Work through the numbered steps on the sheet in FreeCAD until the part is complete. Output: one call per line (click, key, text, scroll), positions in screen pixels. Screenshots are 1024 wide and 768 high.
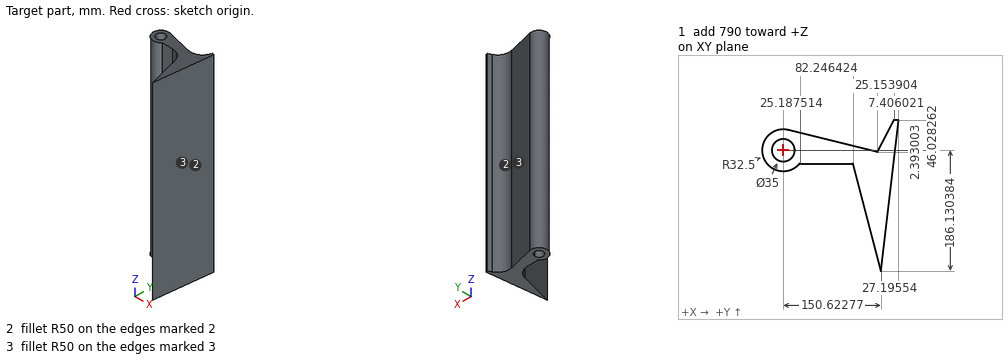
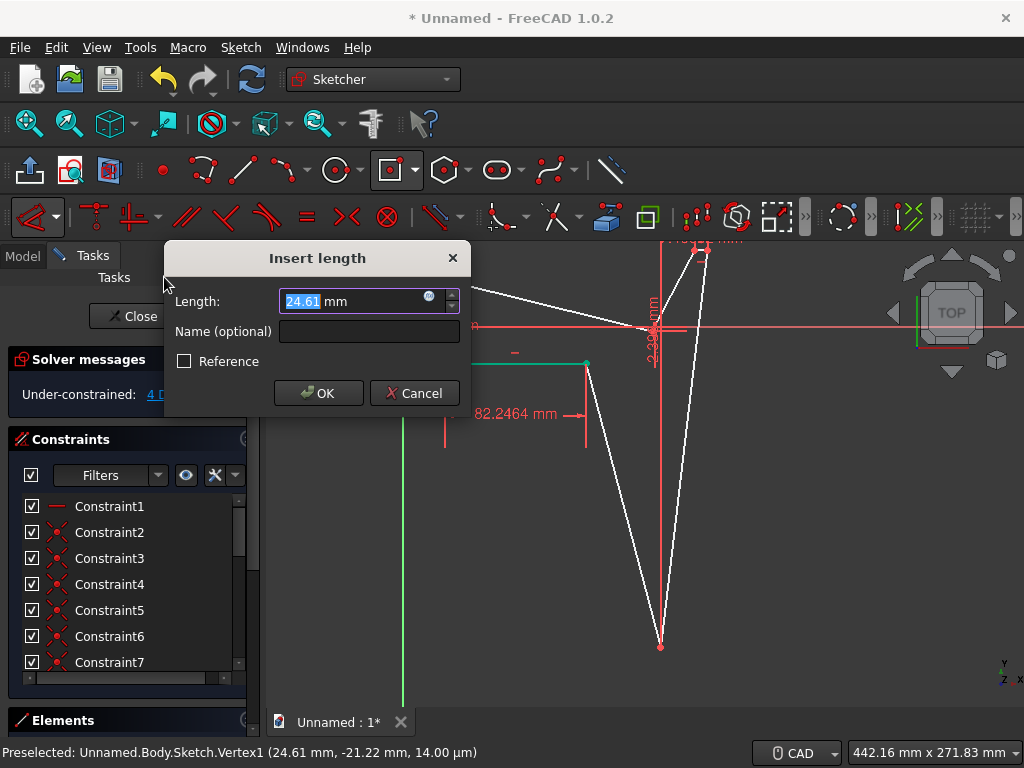
text(25.187514)
key(Return)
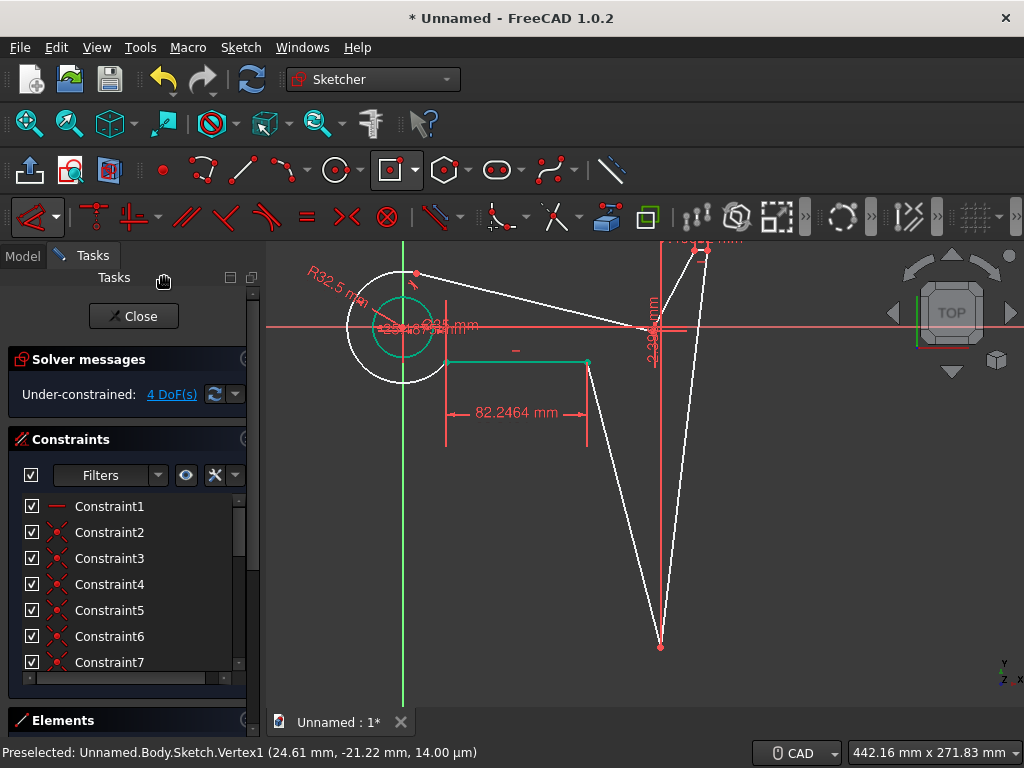
click(661, 647)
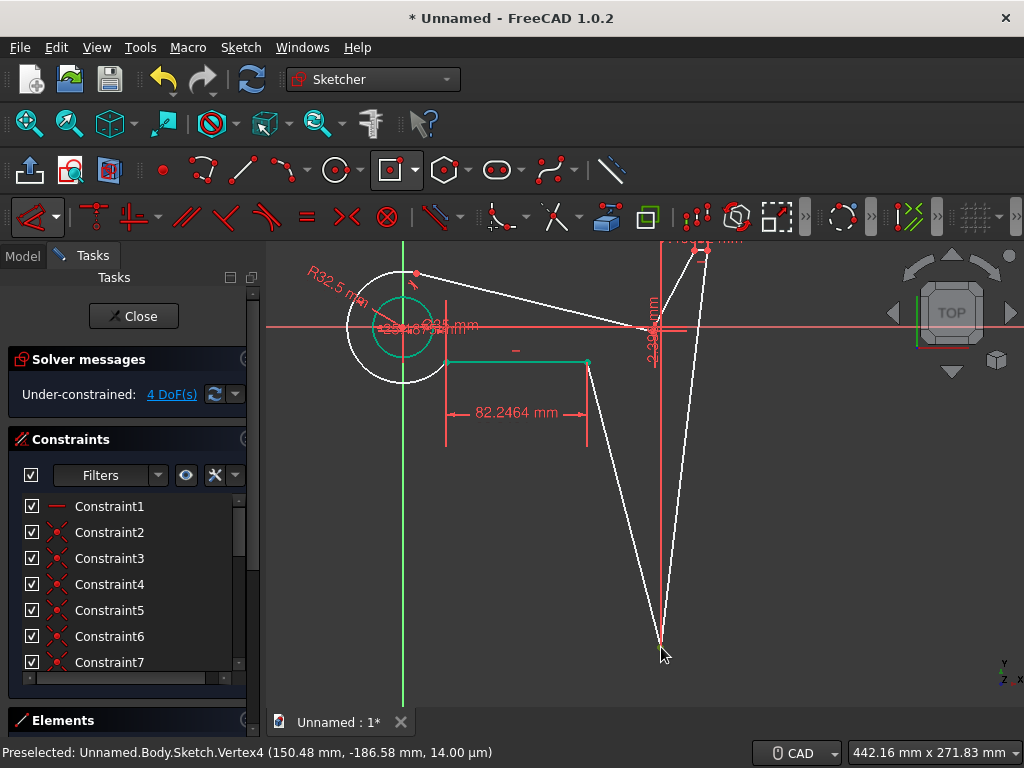
key(l)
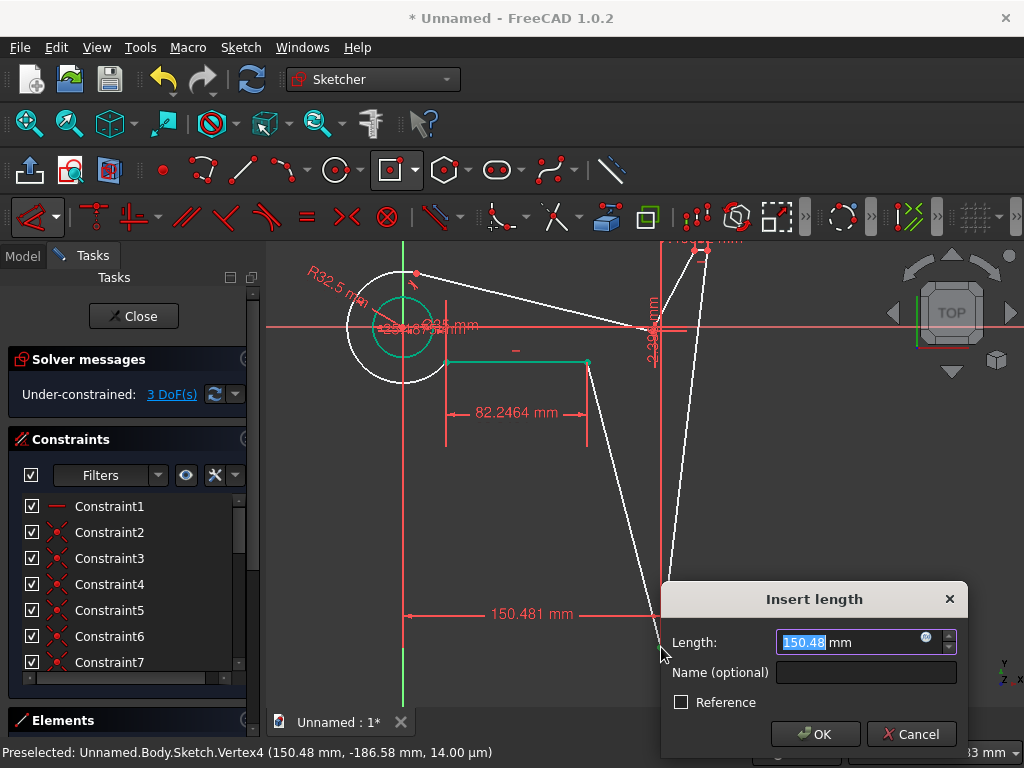
text(150.62277)
key(Return)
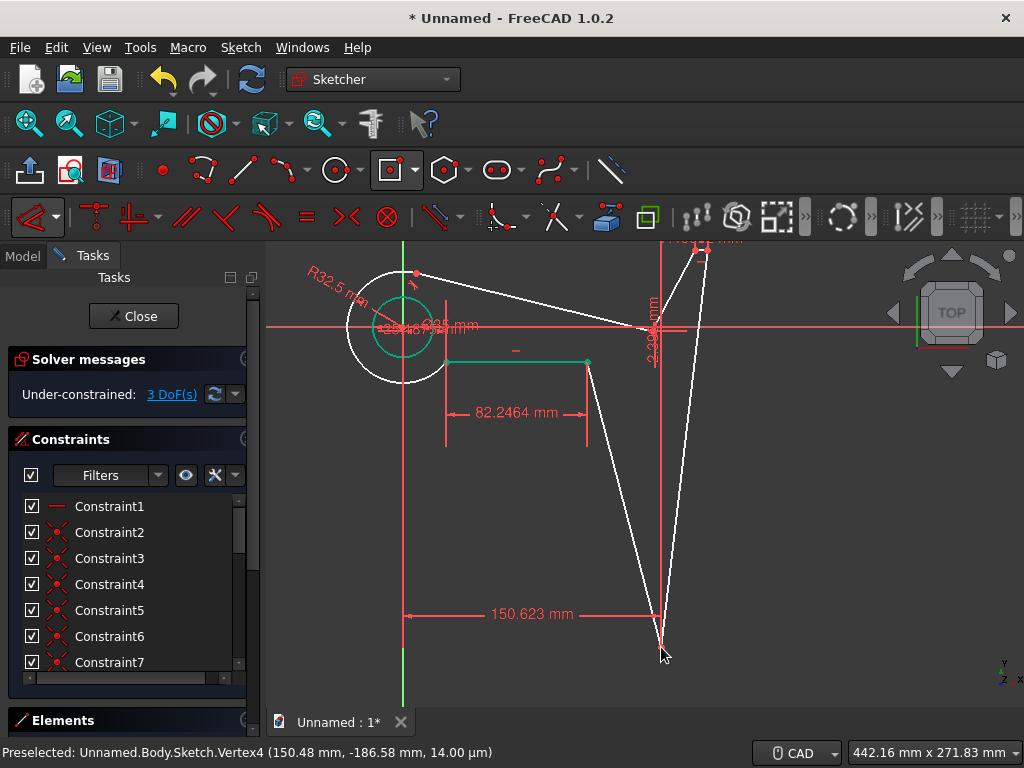
scroll(673, 528, down, 2)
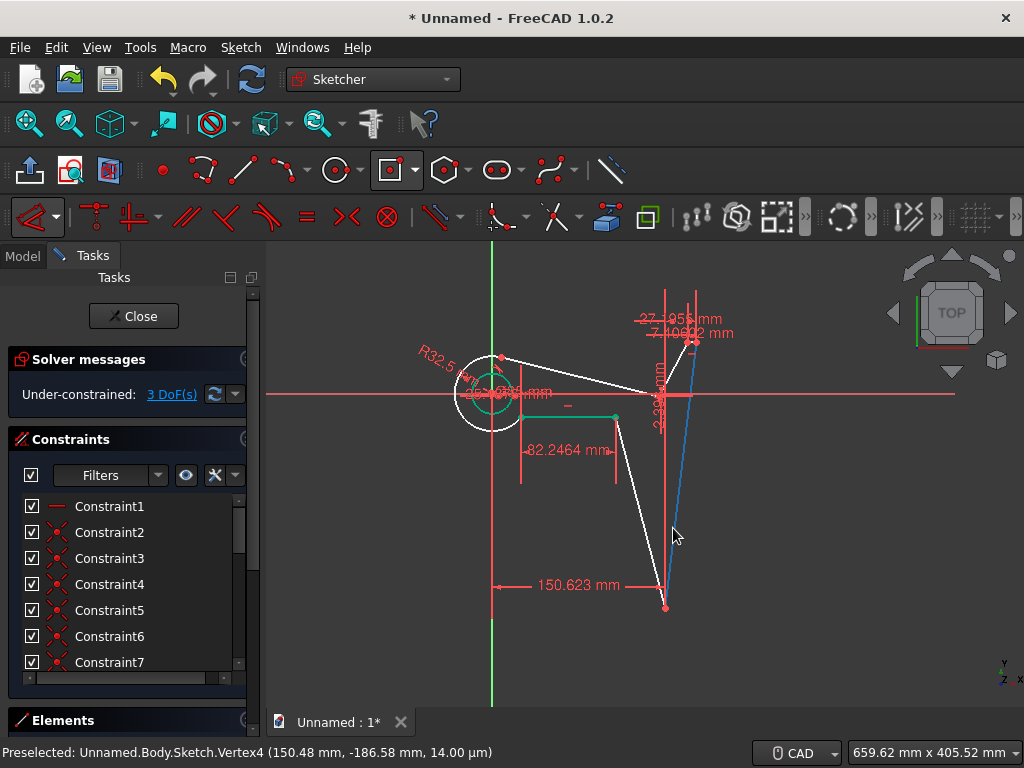
scroll(696, 342, up, 2)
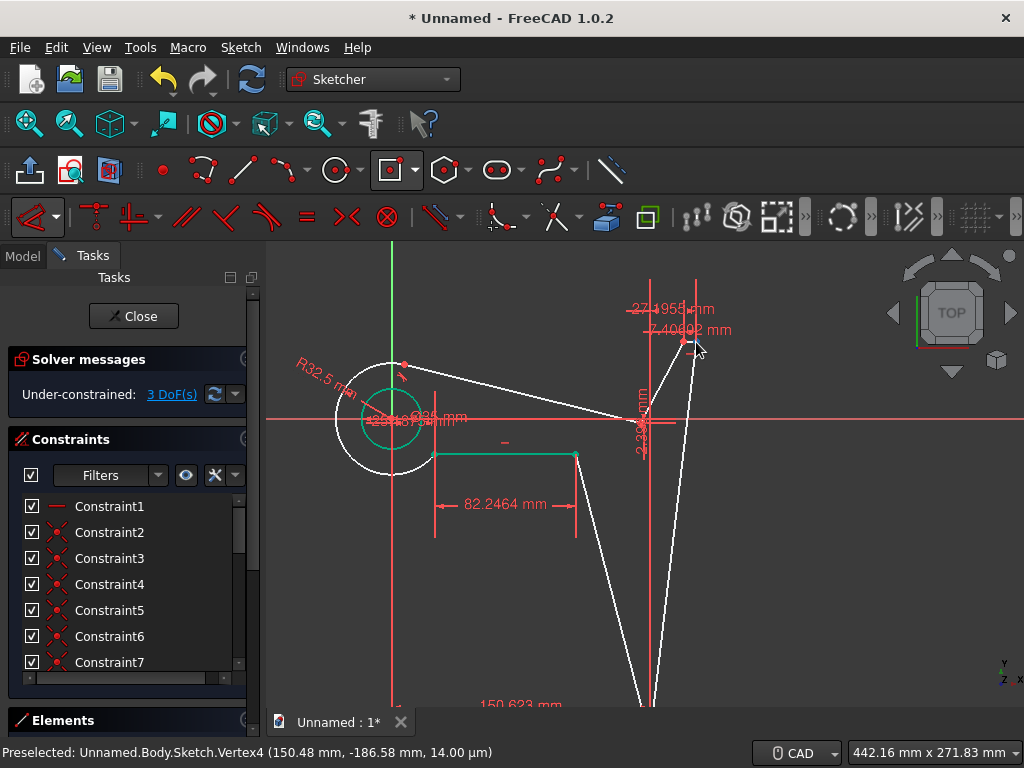
click(696, 342)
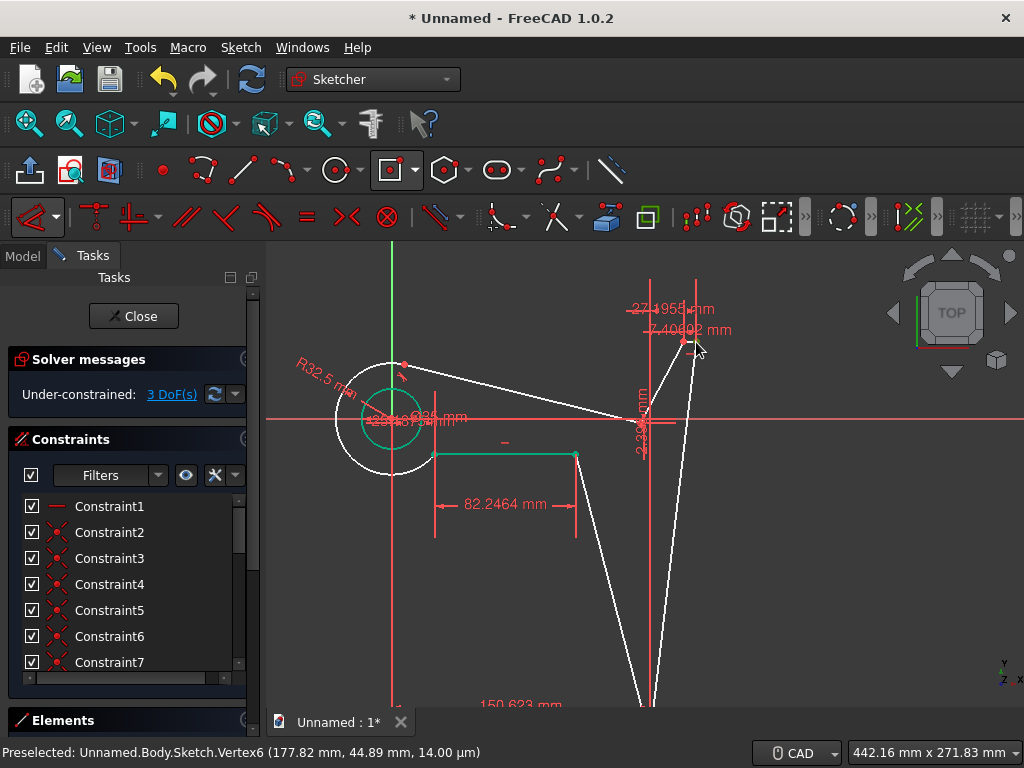
click(58, 218)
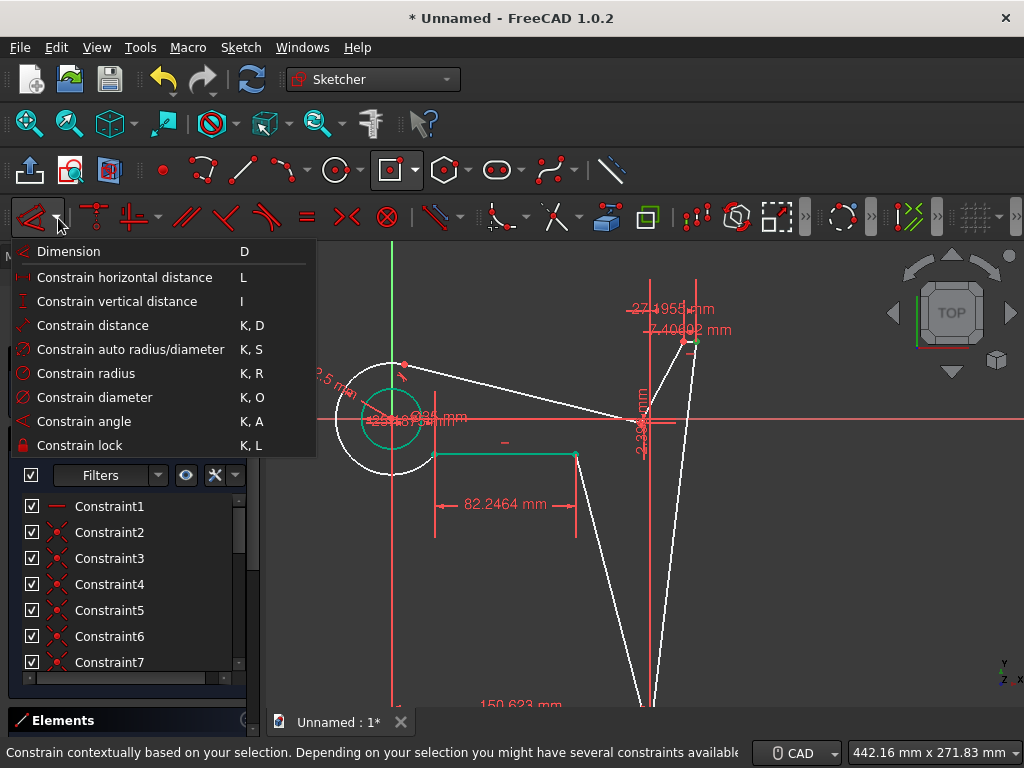
click(164, 301)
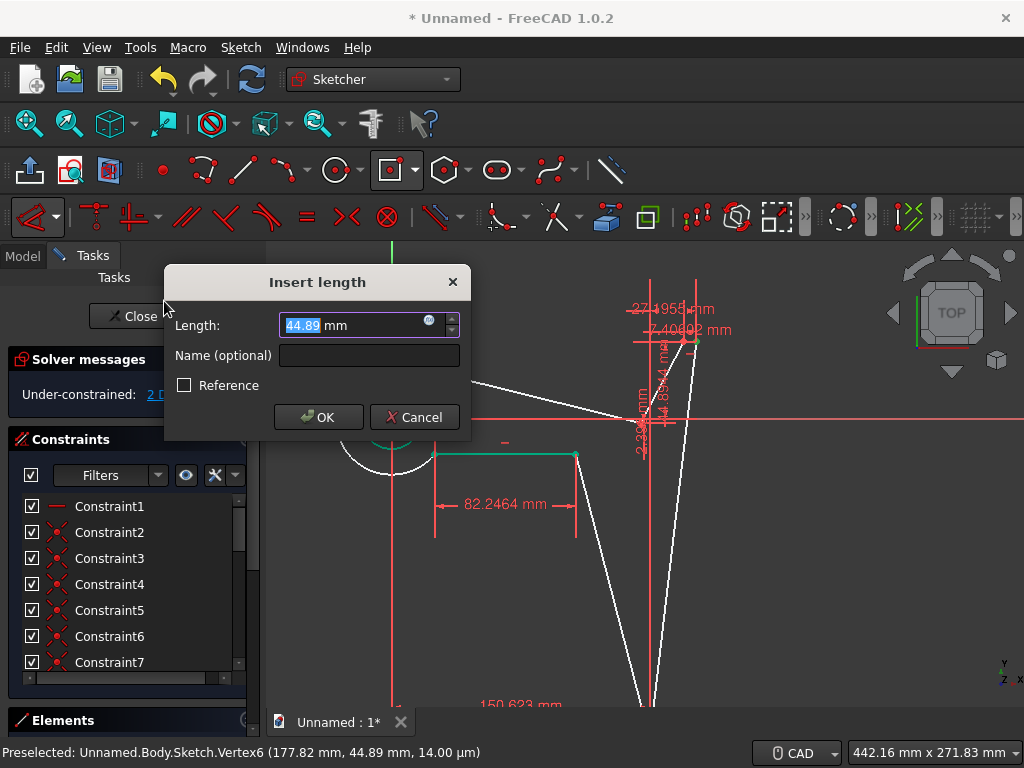
text(46.028262)
key(Return)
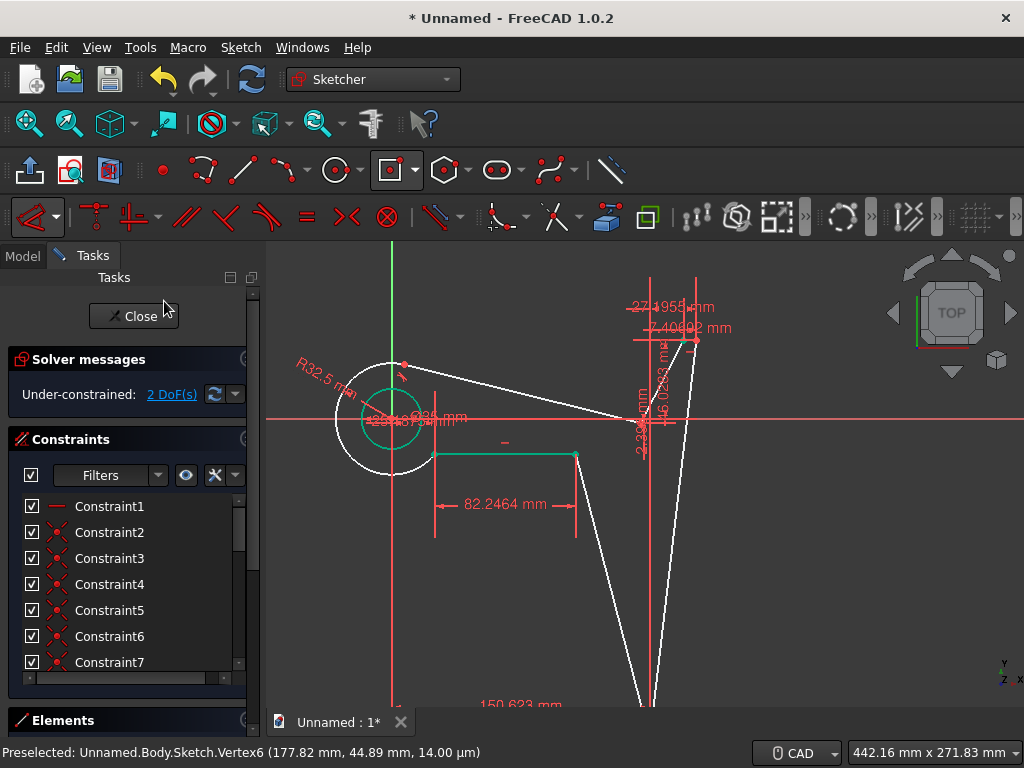
click(654, 398)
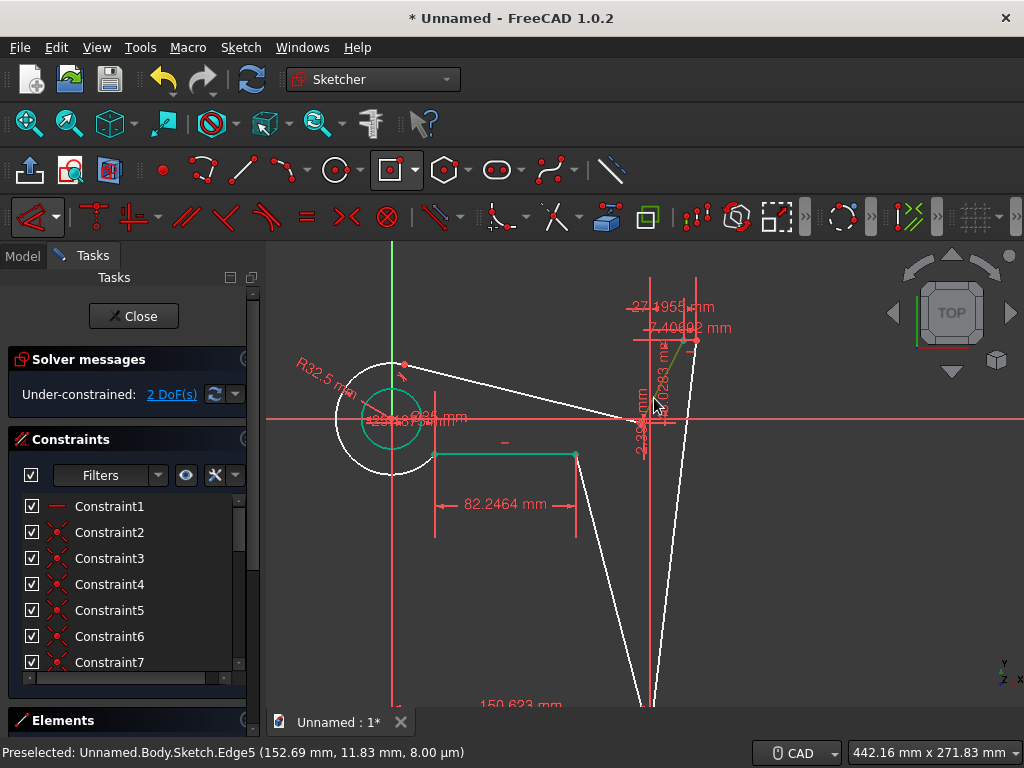
key(l)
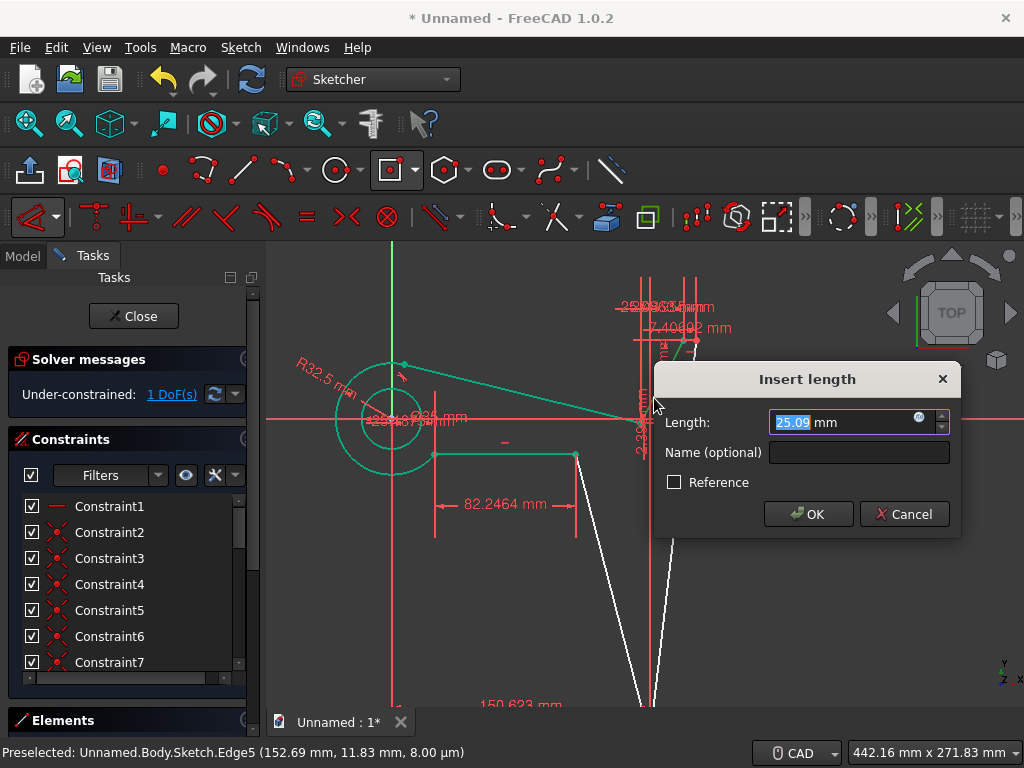
text(25.153904)
key(Return)